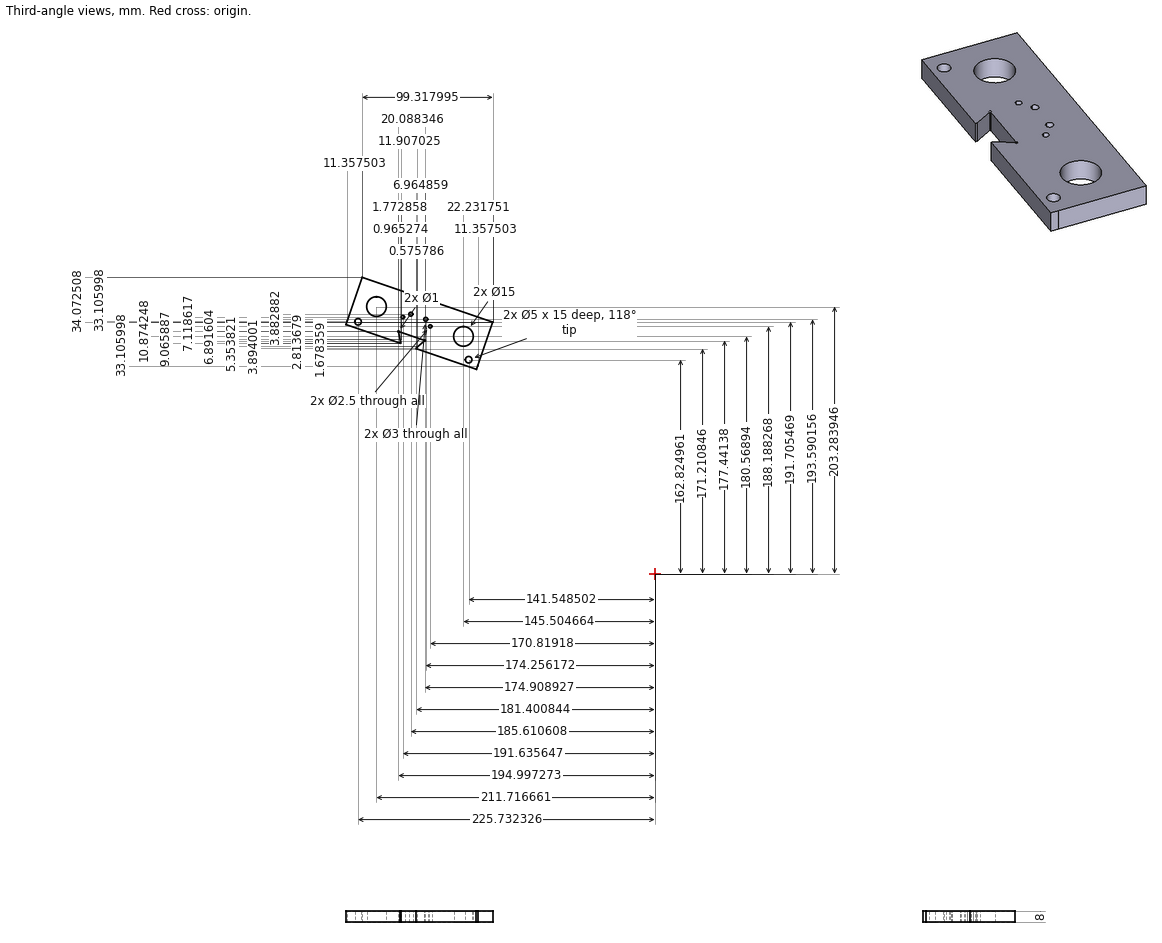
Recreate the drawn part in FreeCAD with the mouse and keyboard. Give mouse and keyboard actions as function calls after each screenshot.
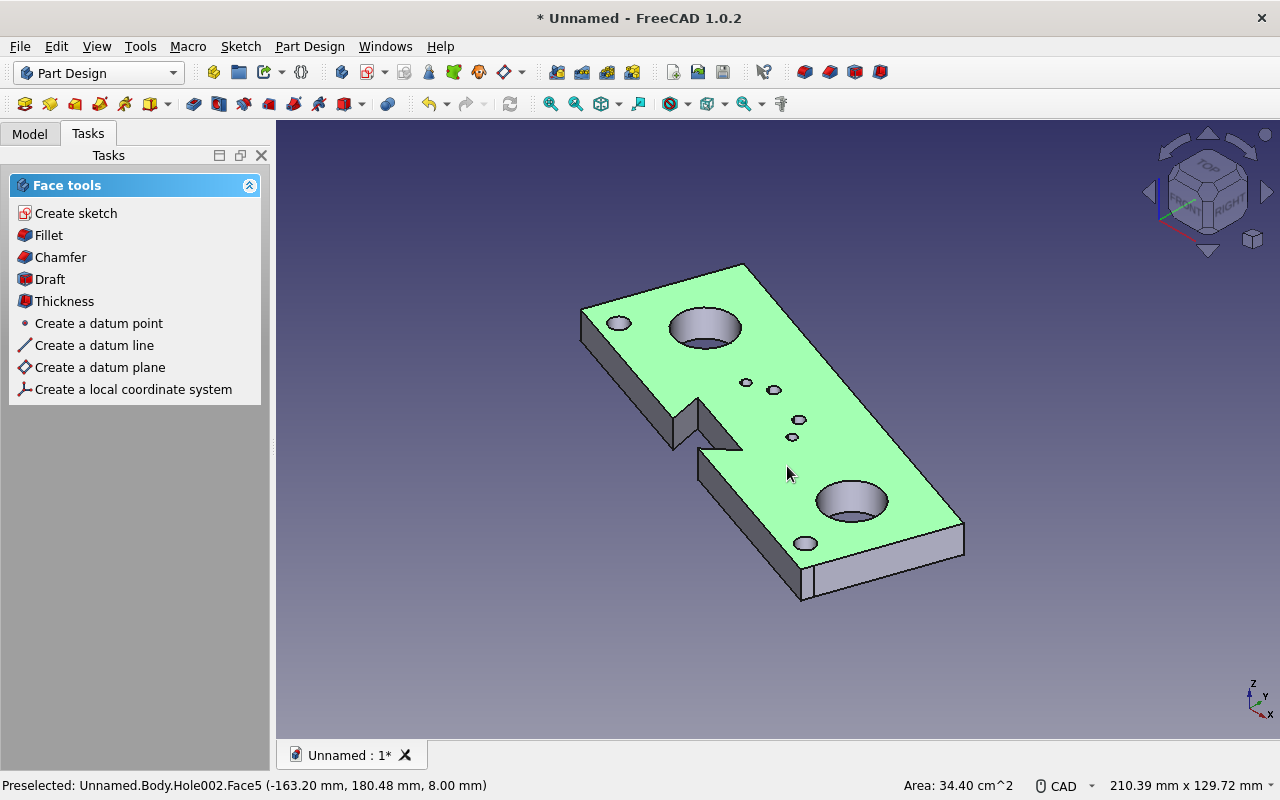
click(366, 72)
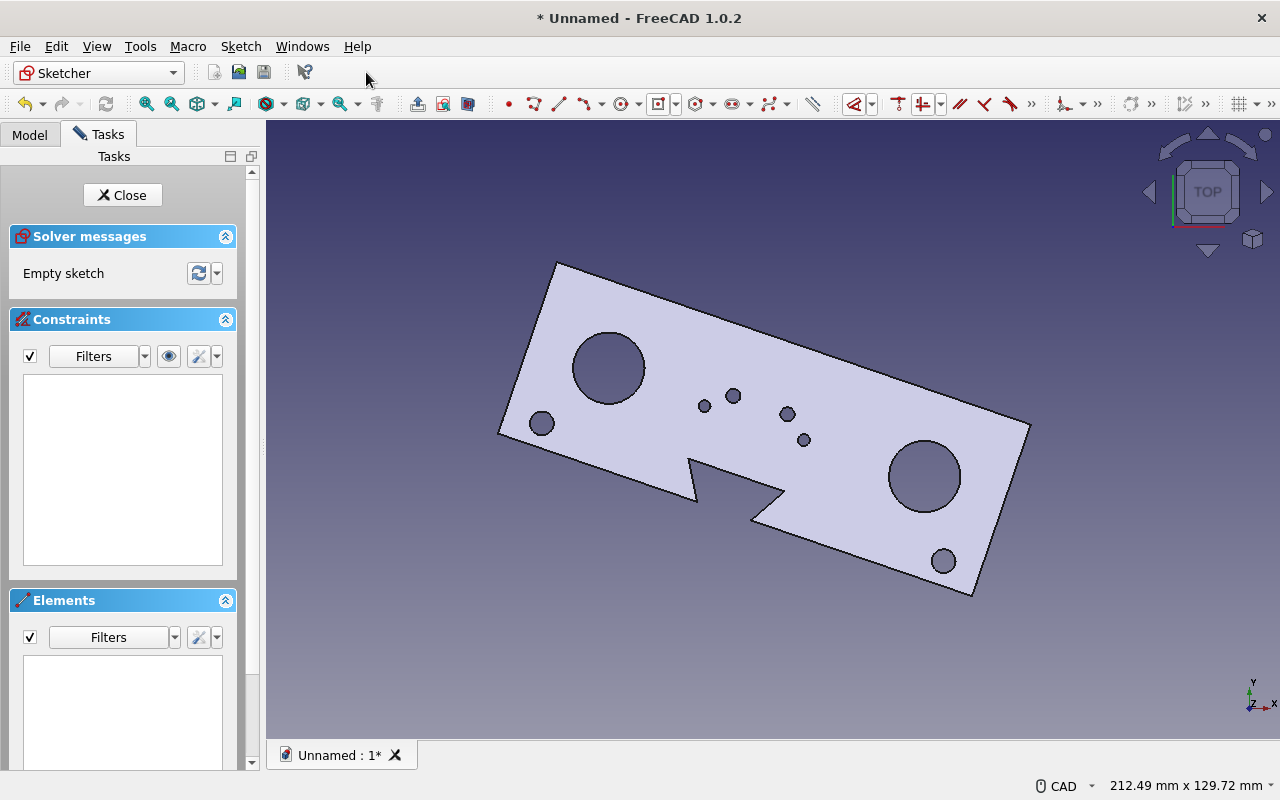
scroll(728, 514, up, 11)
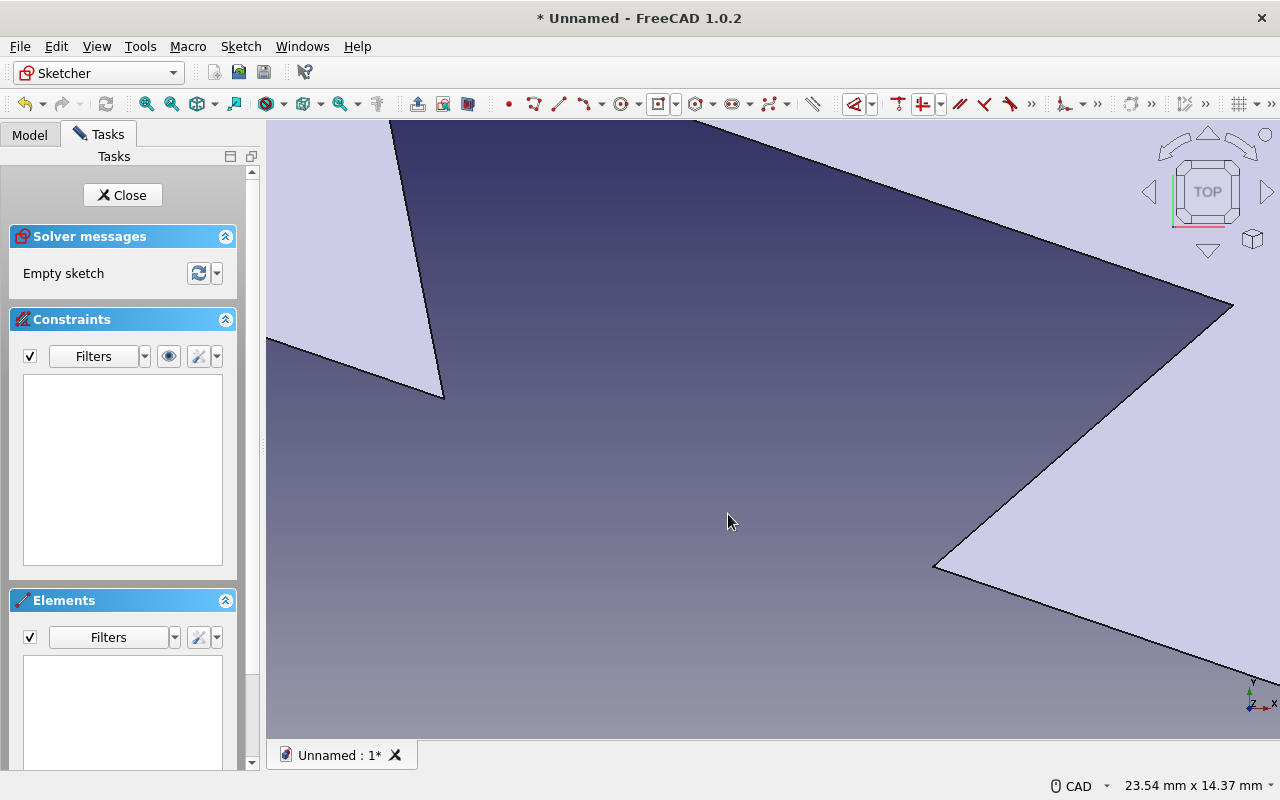
click(534, 104)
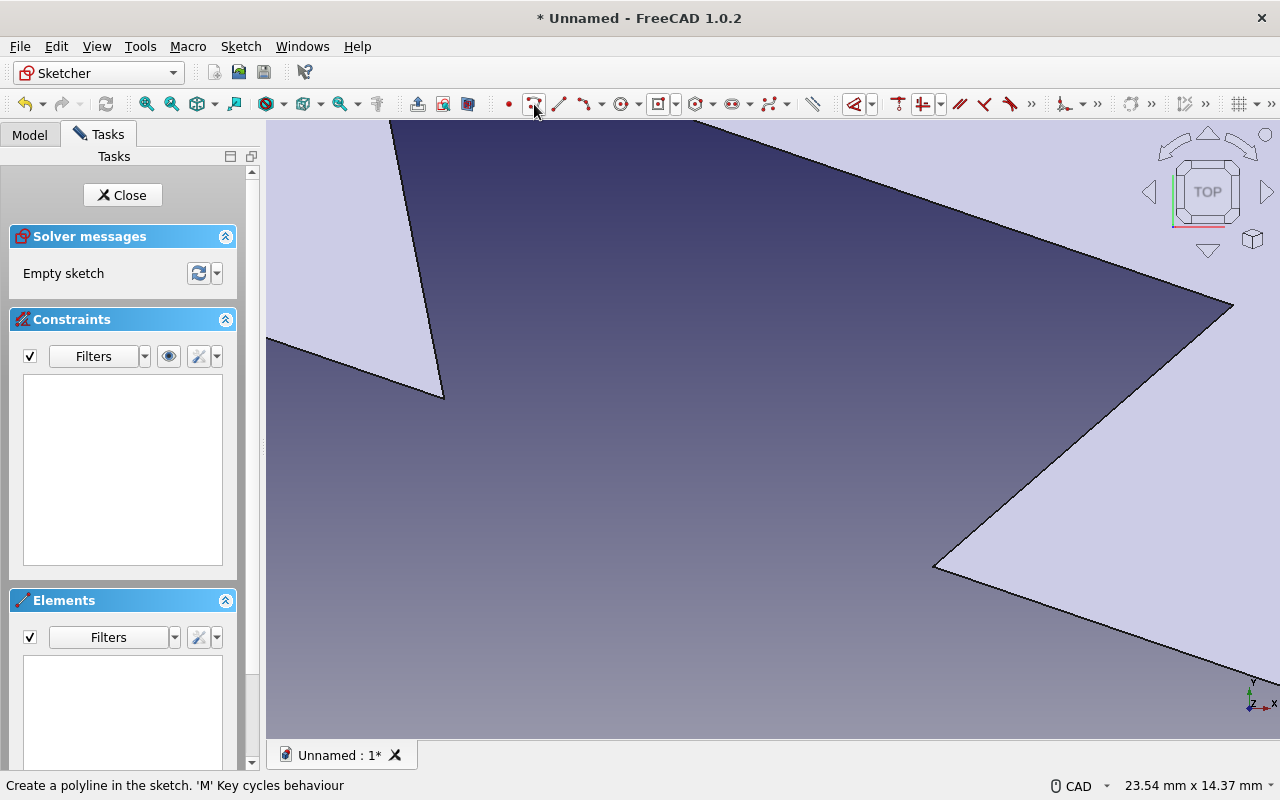
click(953, 574)
click(978, 501)
click(465, 271)
click(424, 392)
click(953, 575)
key(Escape)
key(Escape)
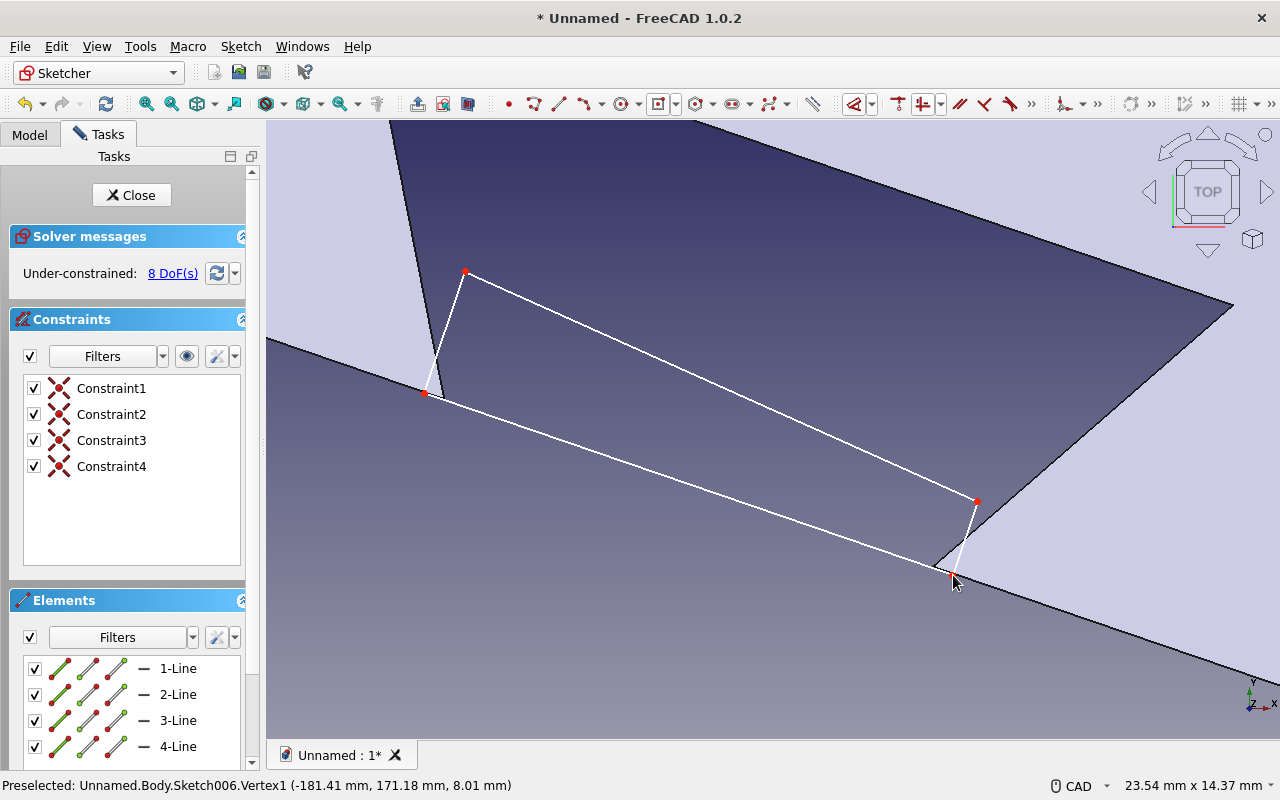
scroll(961, 553, up, 3)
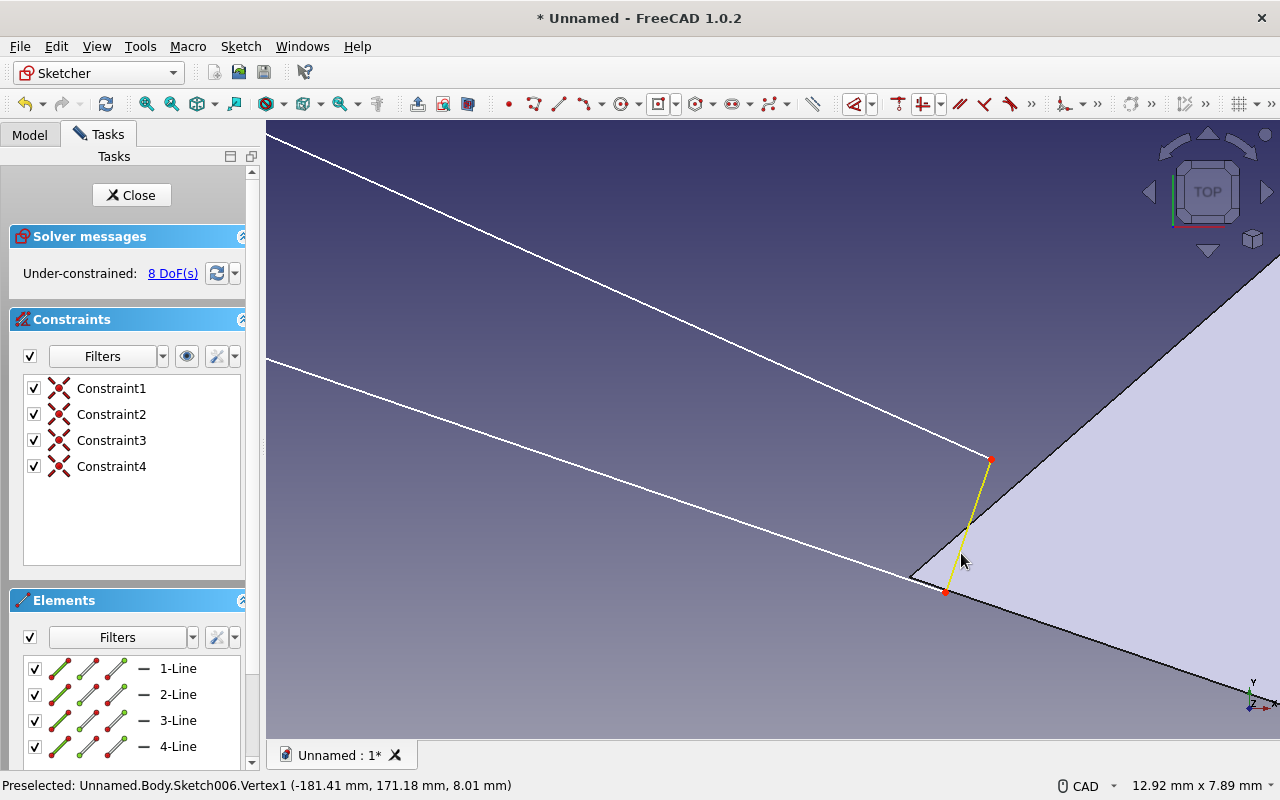
click(960, 553)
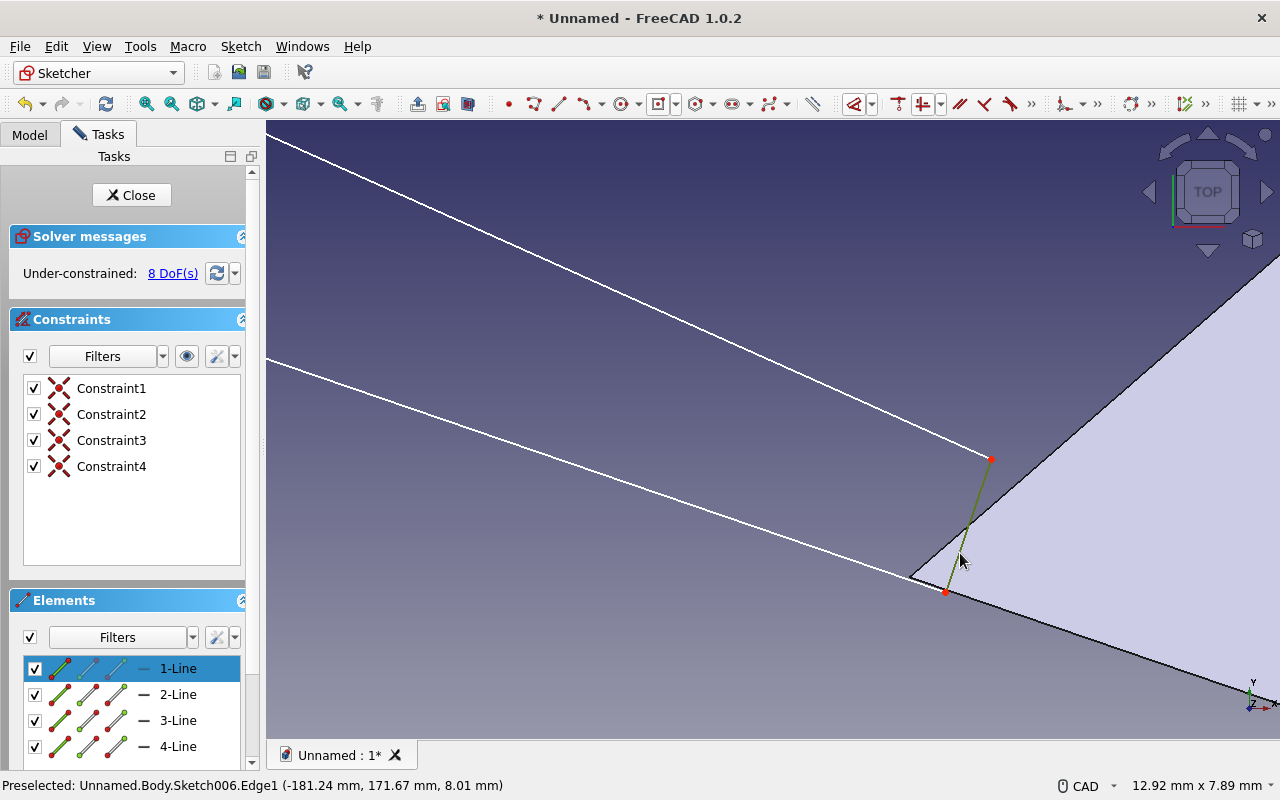
key(l)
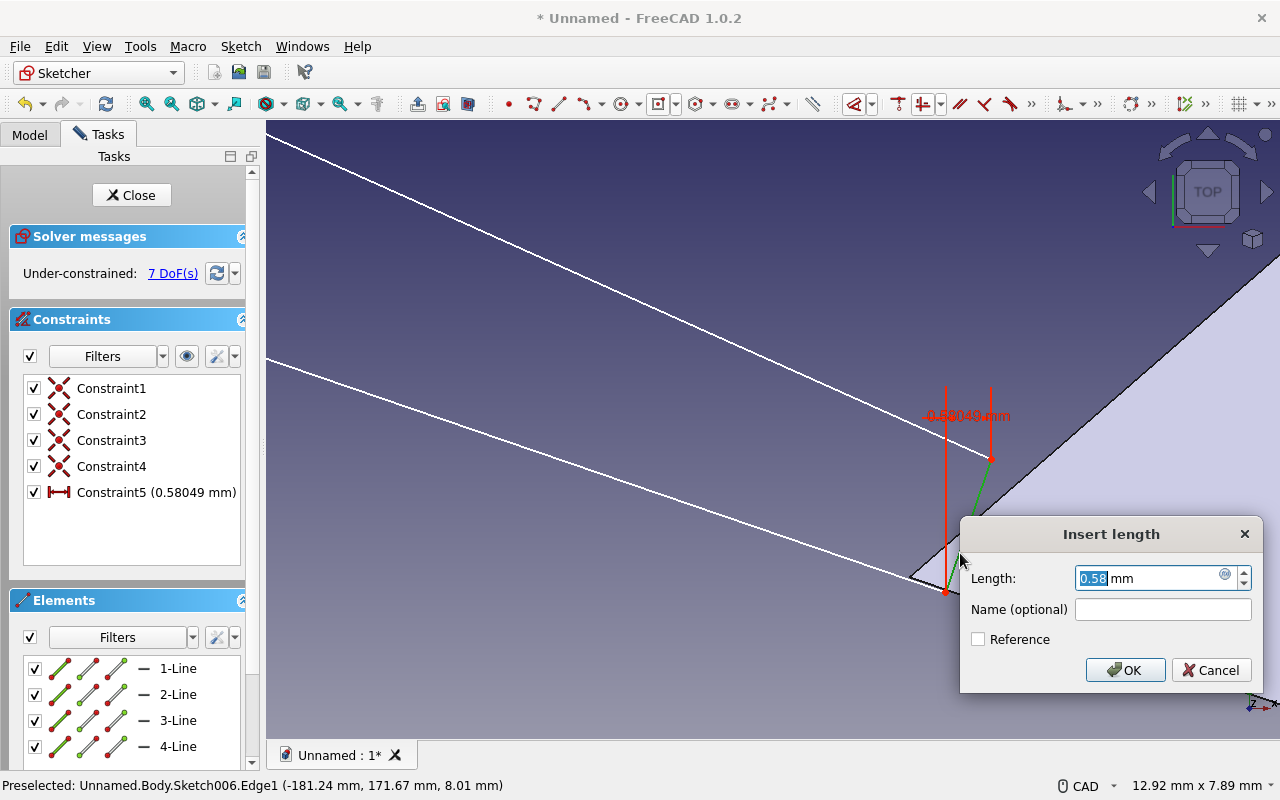
text(0.575786)
key(Return)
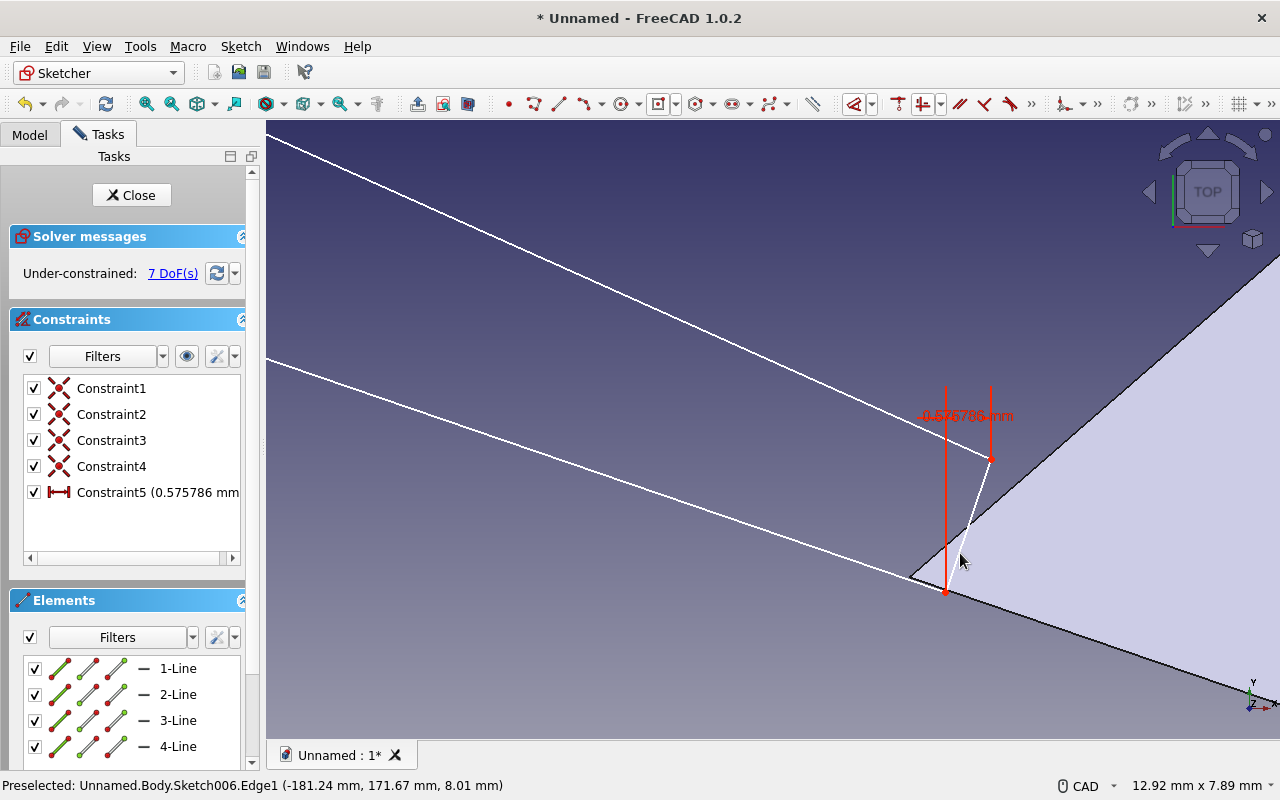
click(959, 553)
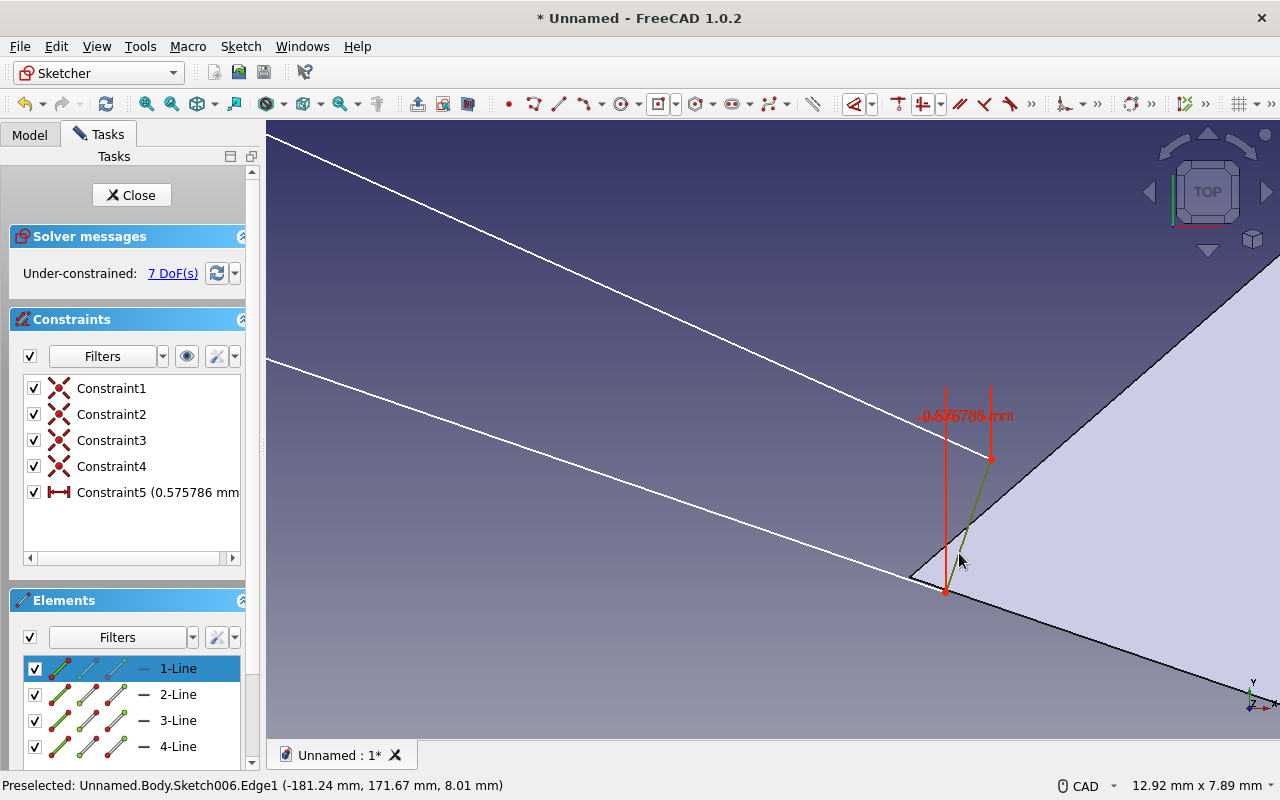
click(872, 104)